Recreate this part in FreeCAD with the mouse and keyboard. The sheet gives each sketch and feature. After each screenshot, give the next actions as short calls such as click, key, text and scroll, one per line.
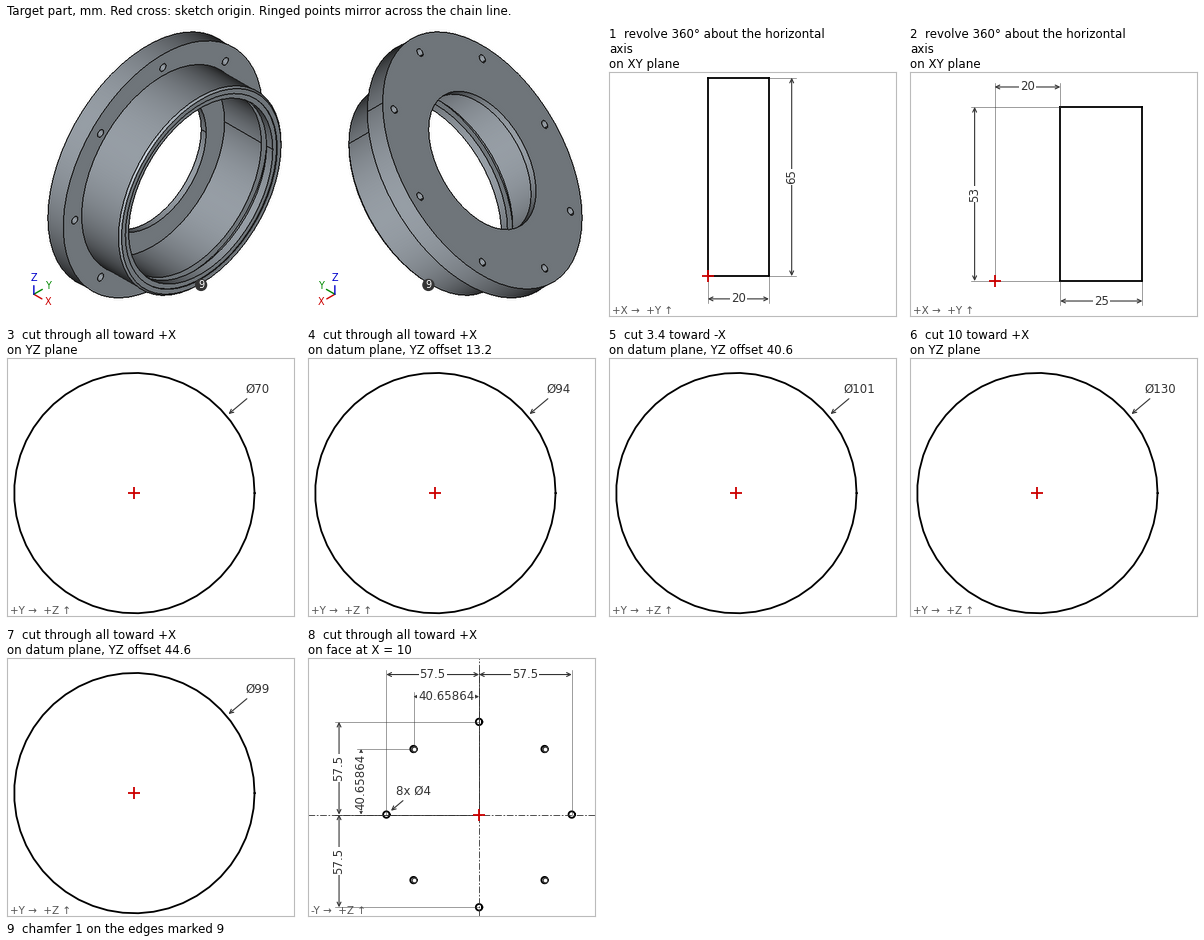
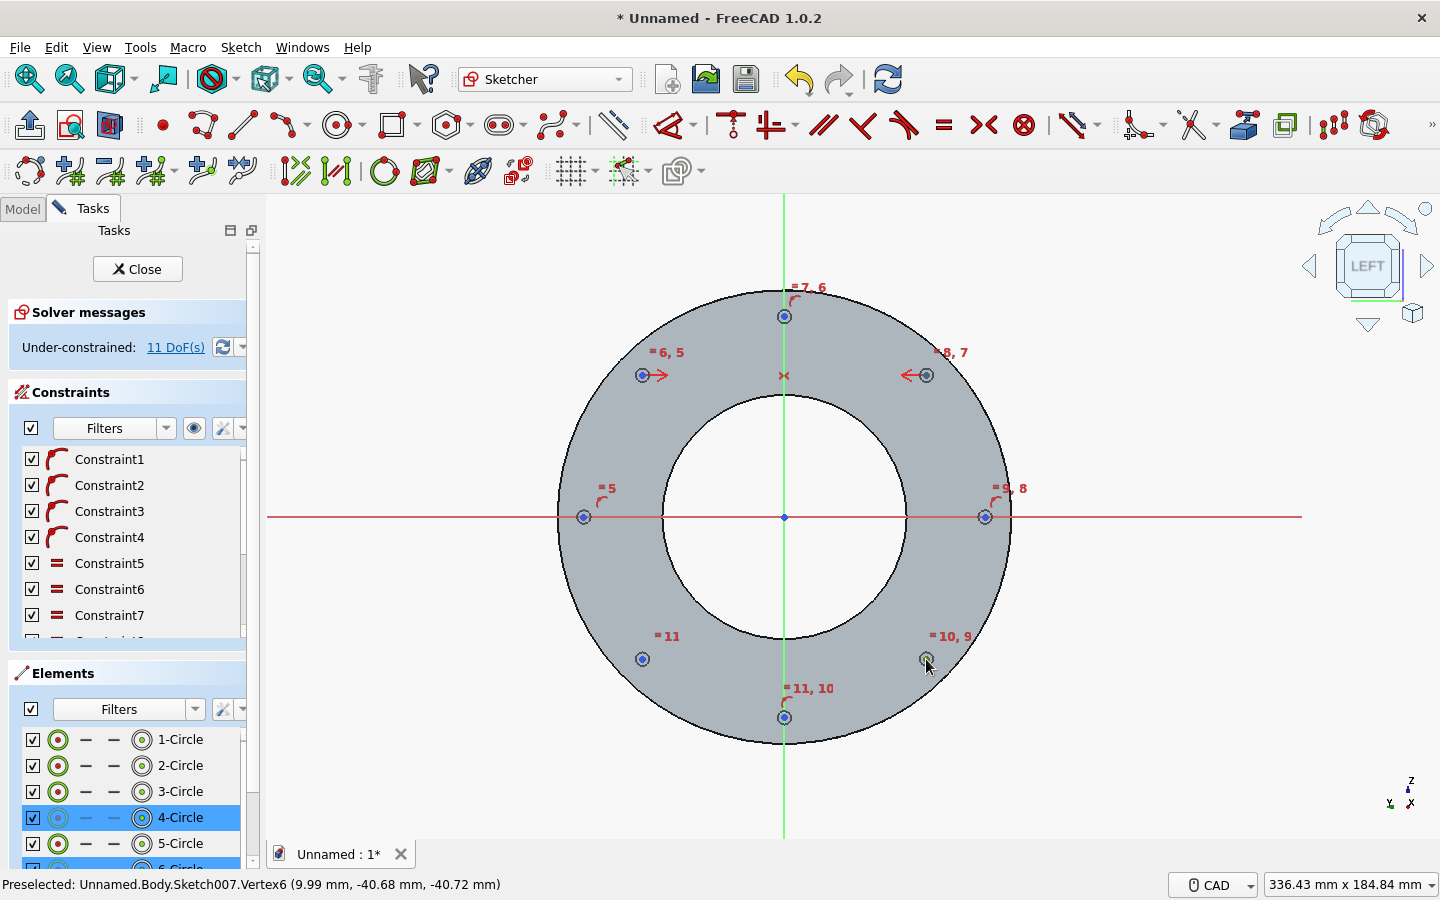
click(364, 517)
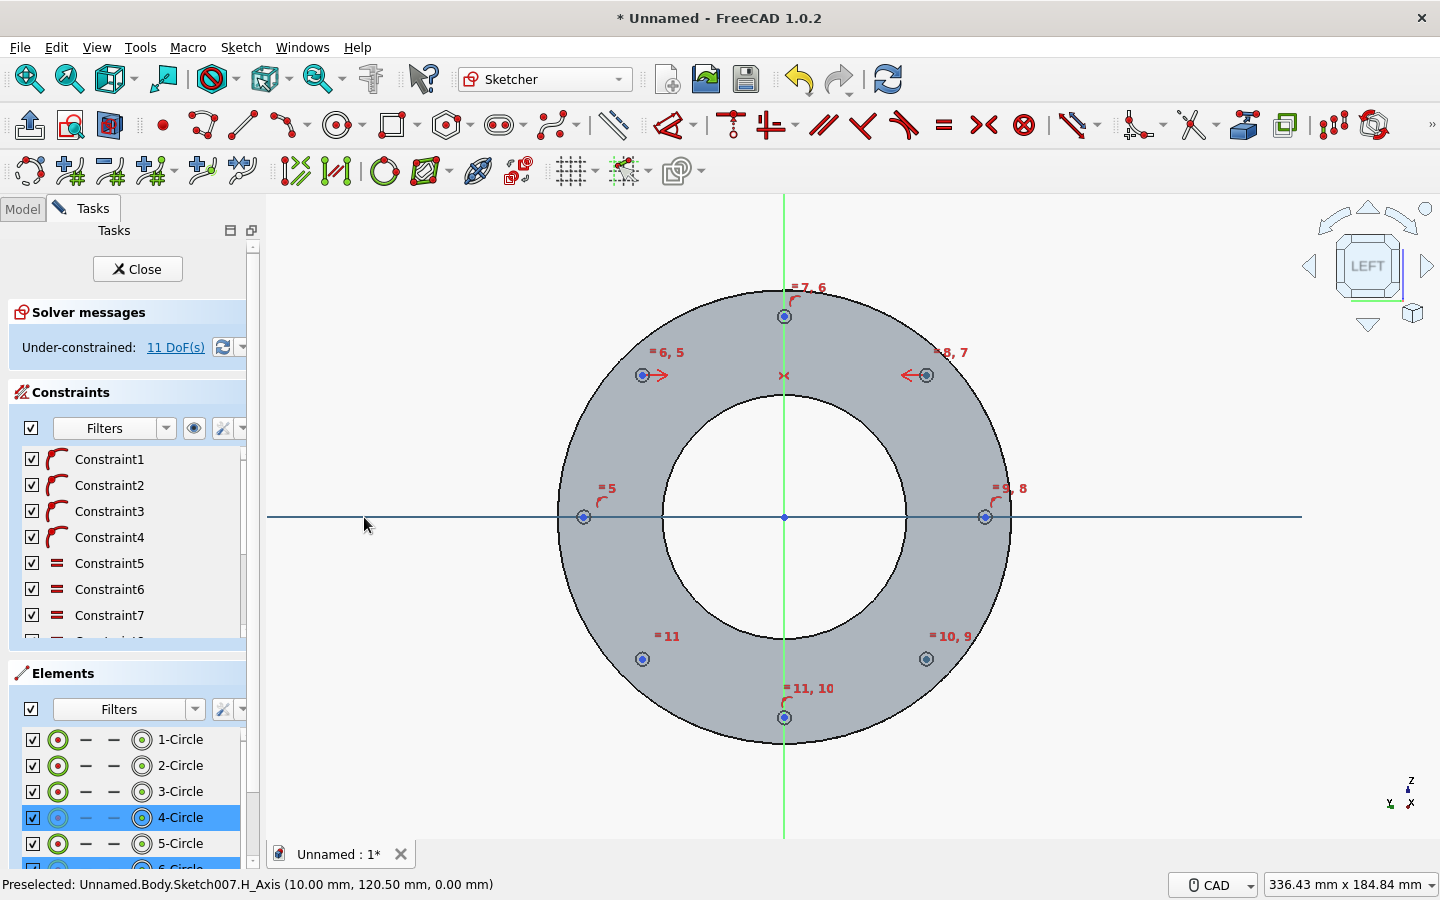
click(984, 126)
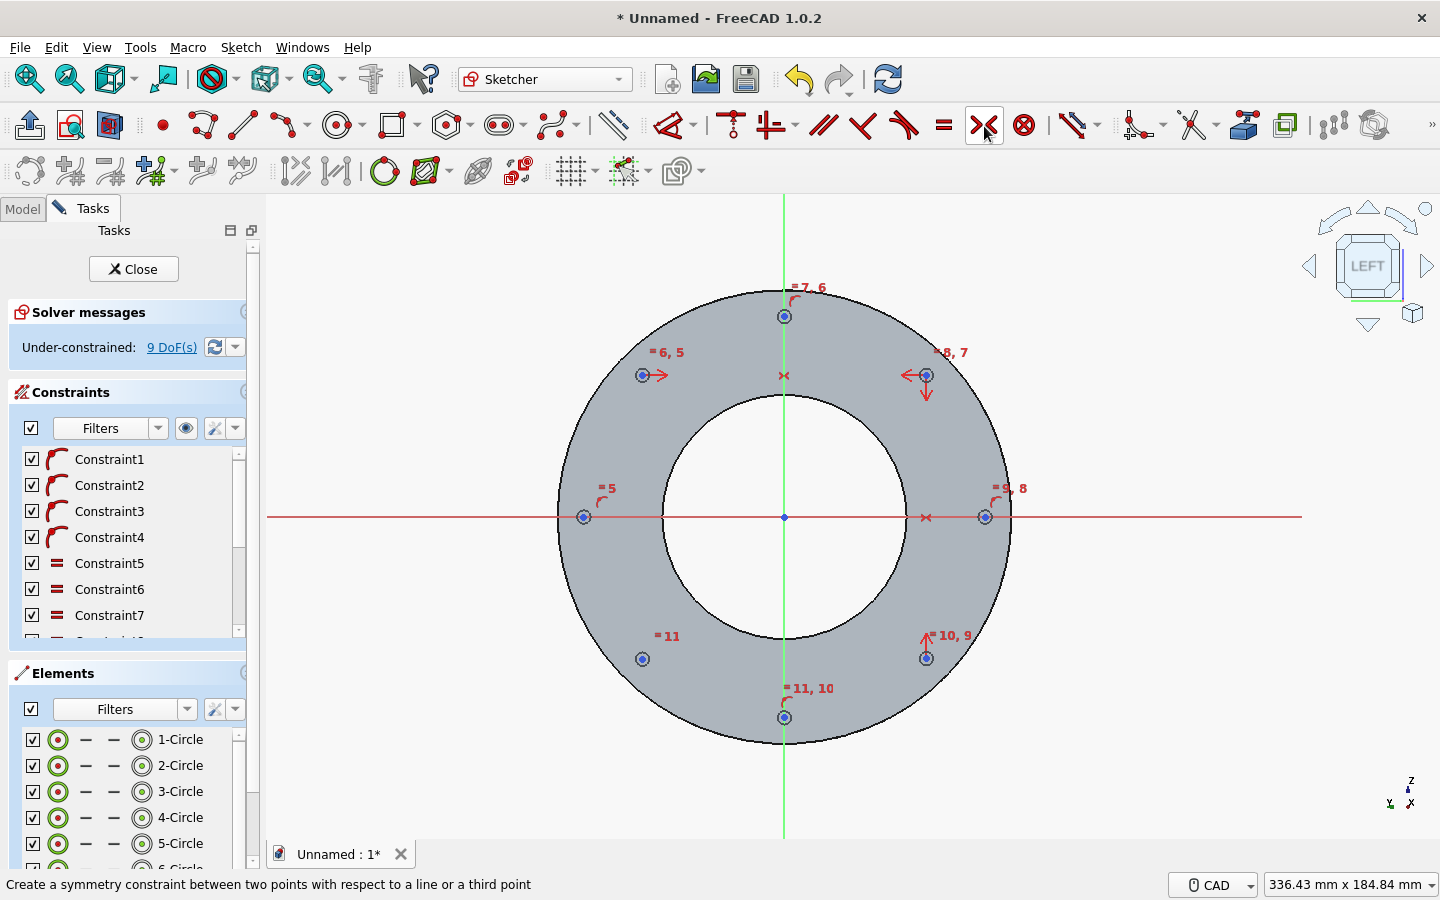
click(643, 375)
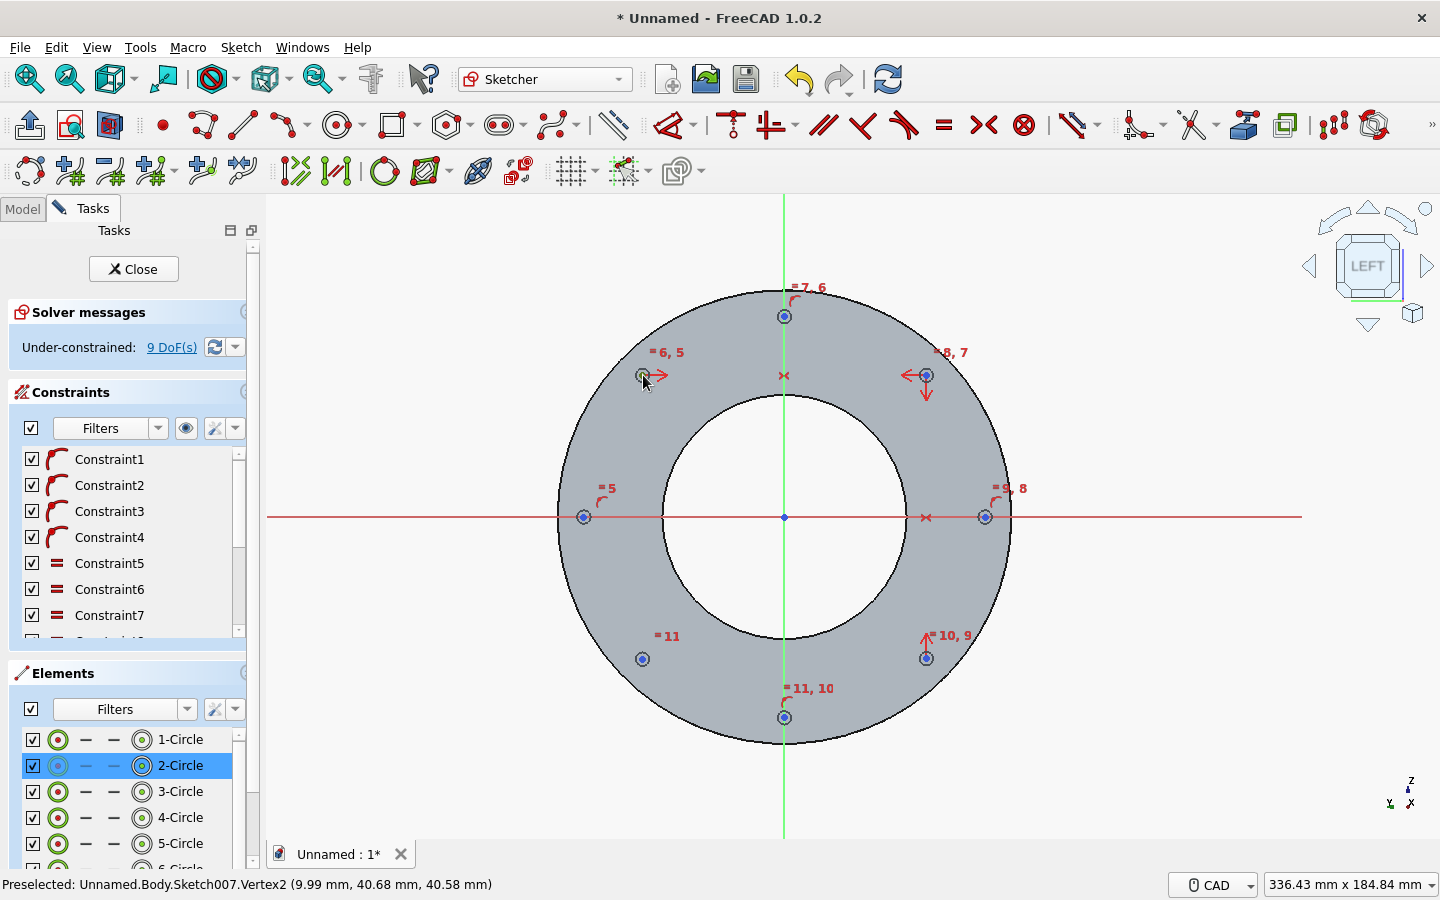
click(642, 659)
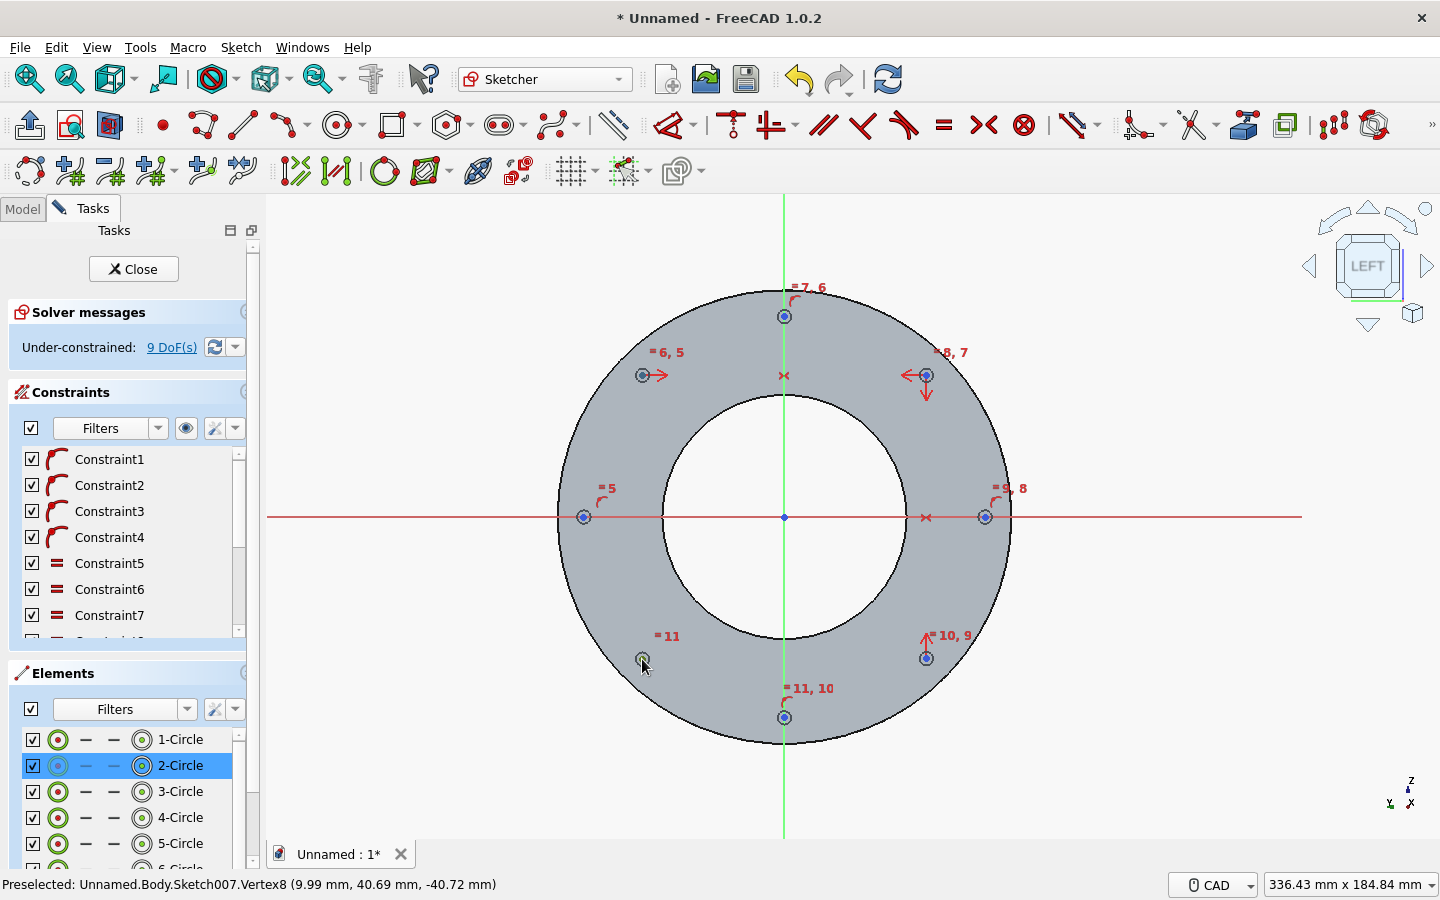
click(364, 517)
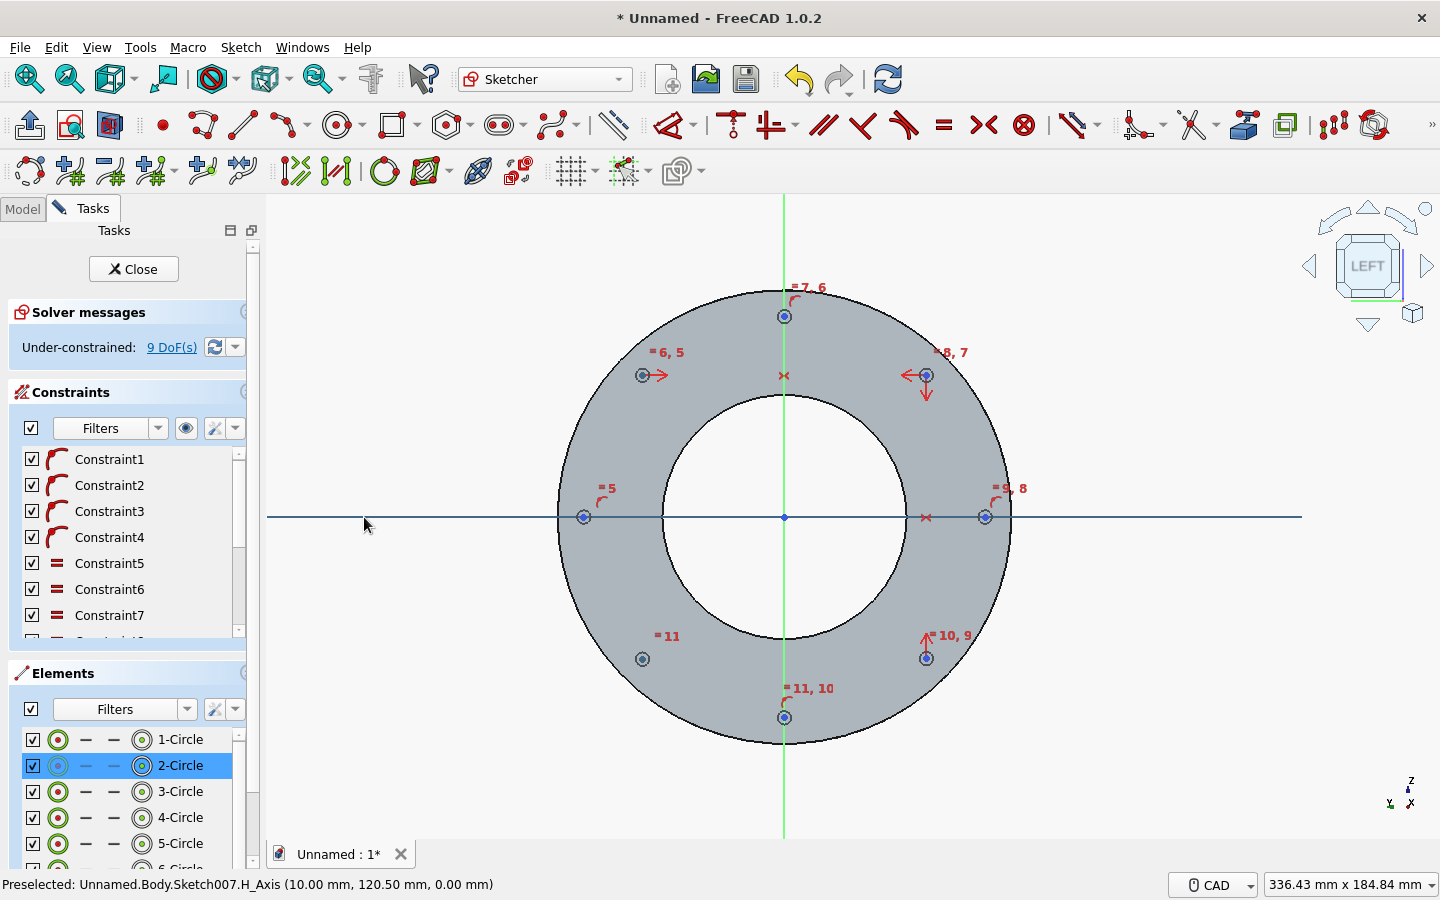
click(984, 126)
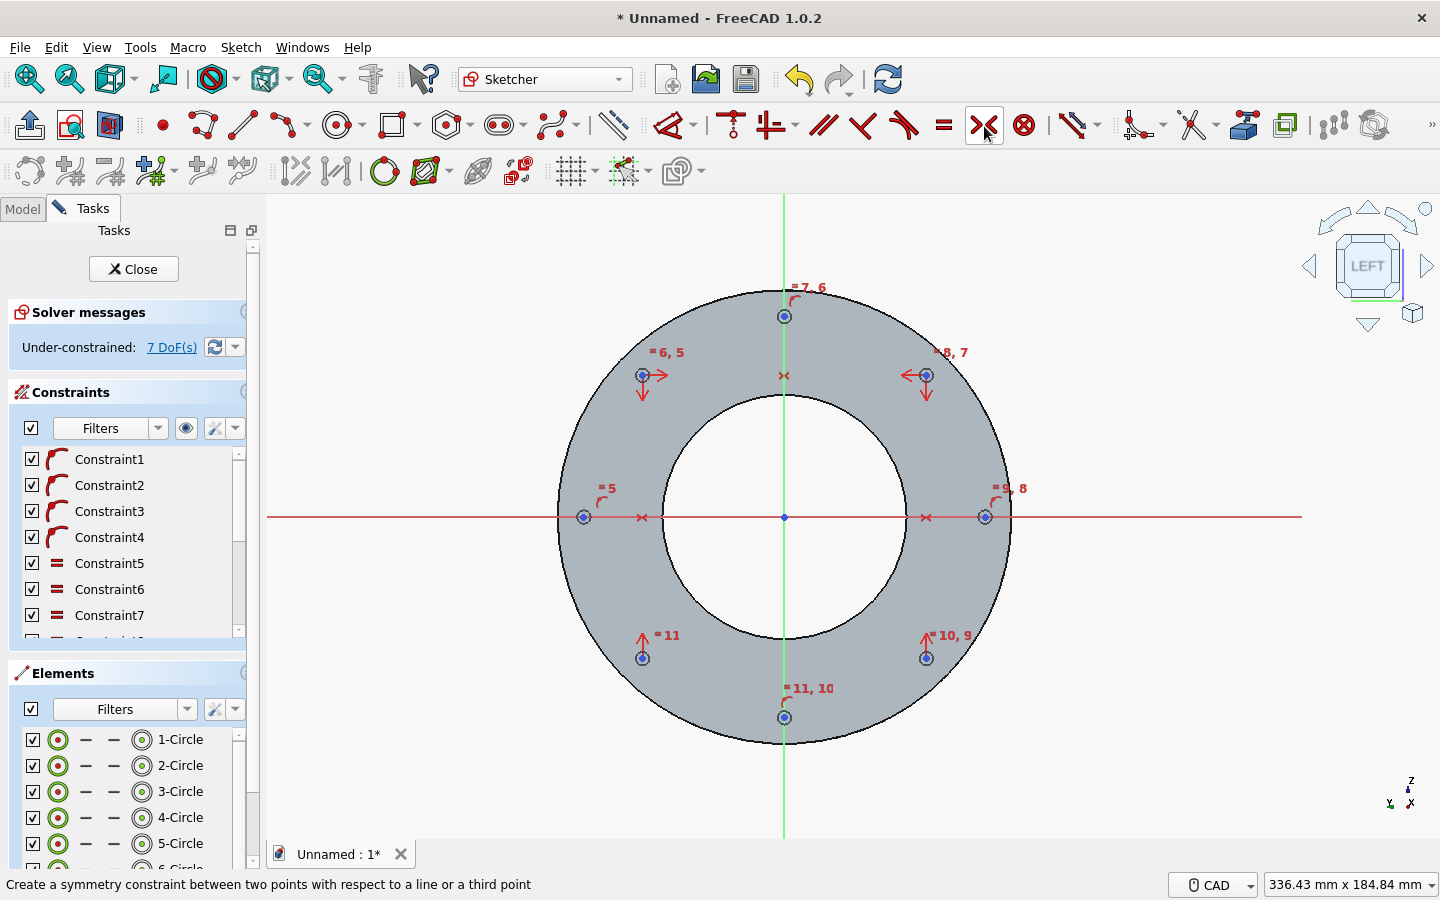
click(668, 126)